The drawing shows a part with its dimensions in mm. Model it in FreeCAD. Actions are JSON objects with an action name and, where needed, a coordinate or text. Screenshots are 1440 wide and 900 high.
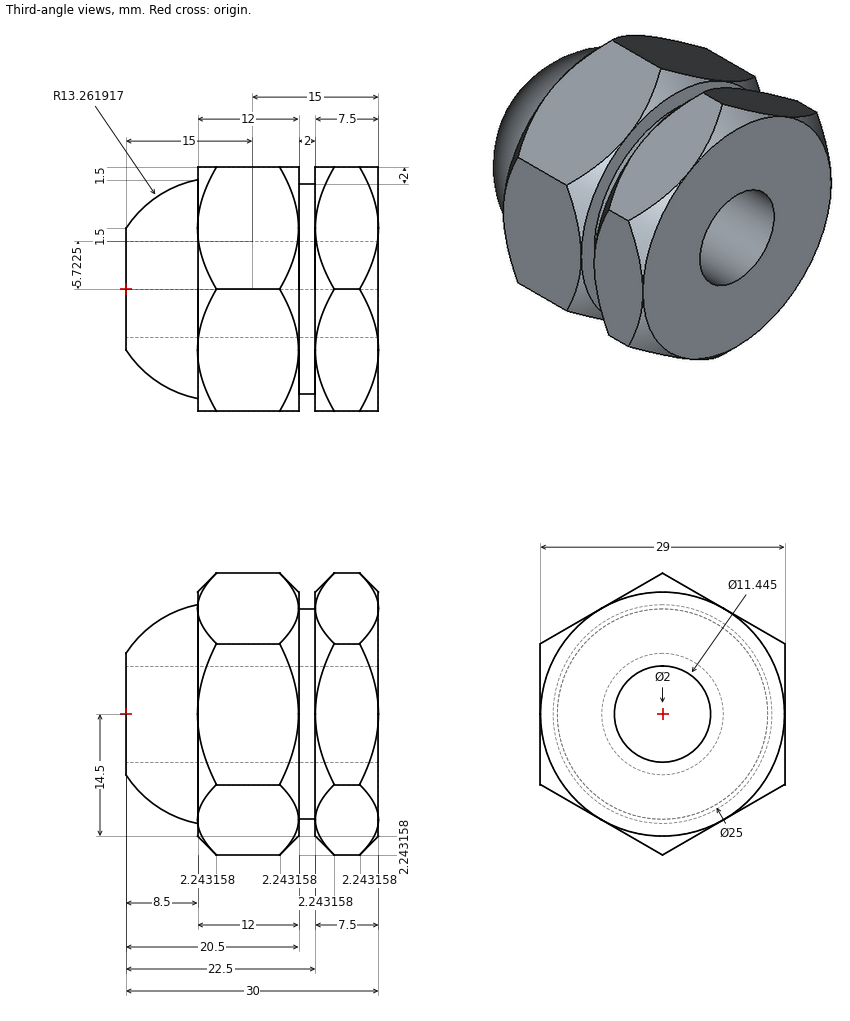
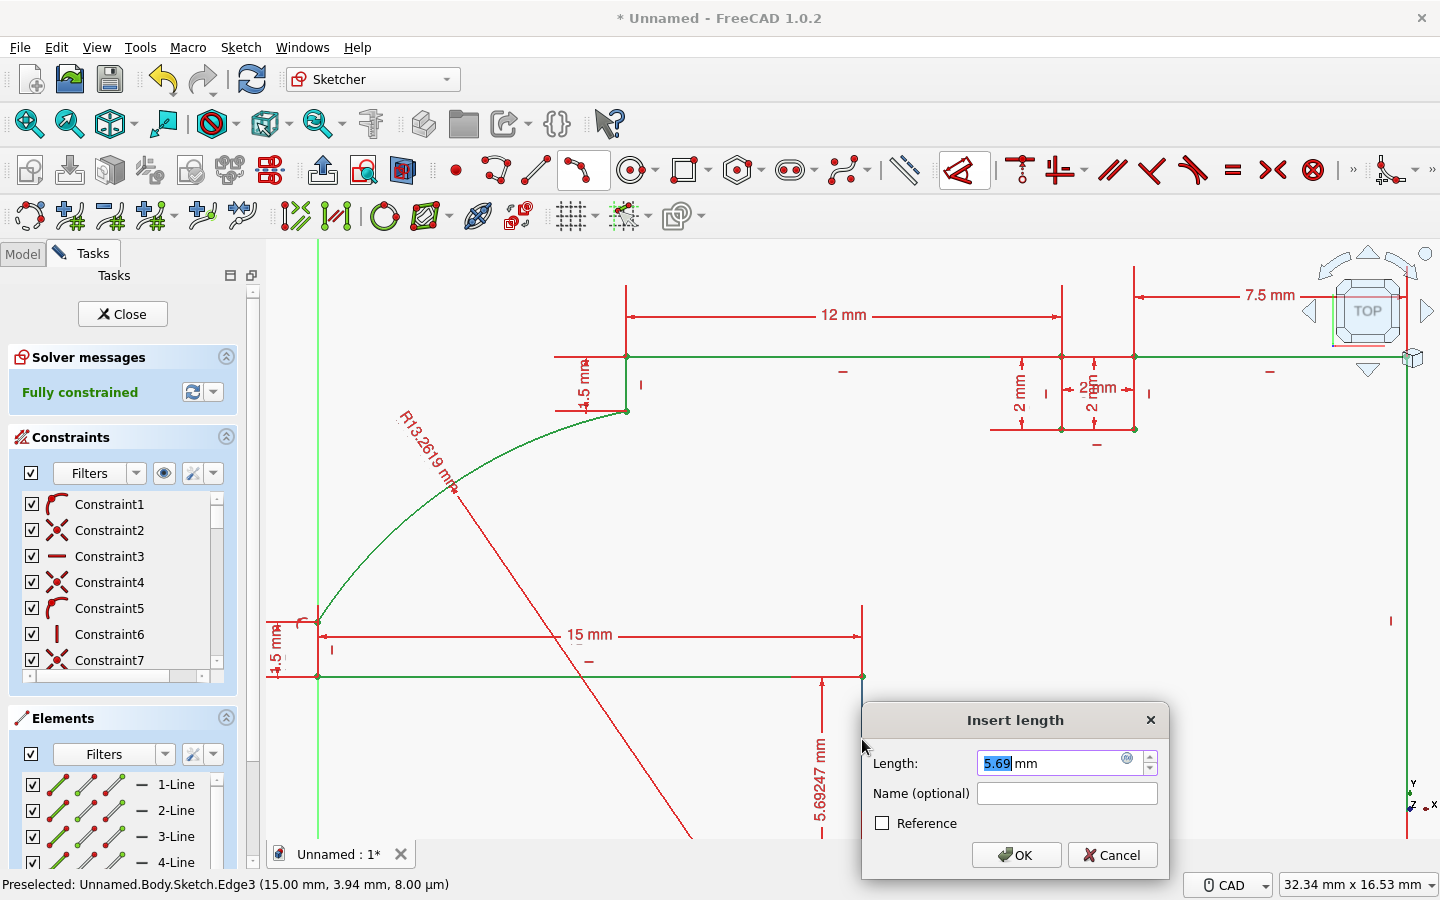
{"action": "type", "text": "5.7225"}
{"action": "key", "text": "Return"}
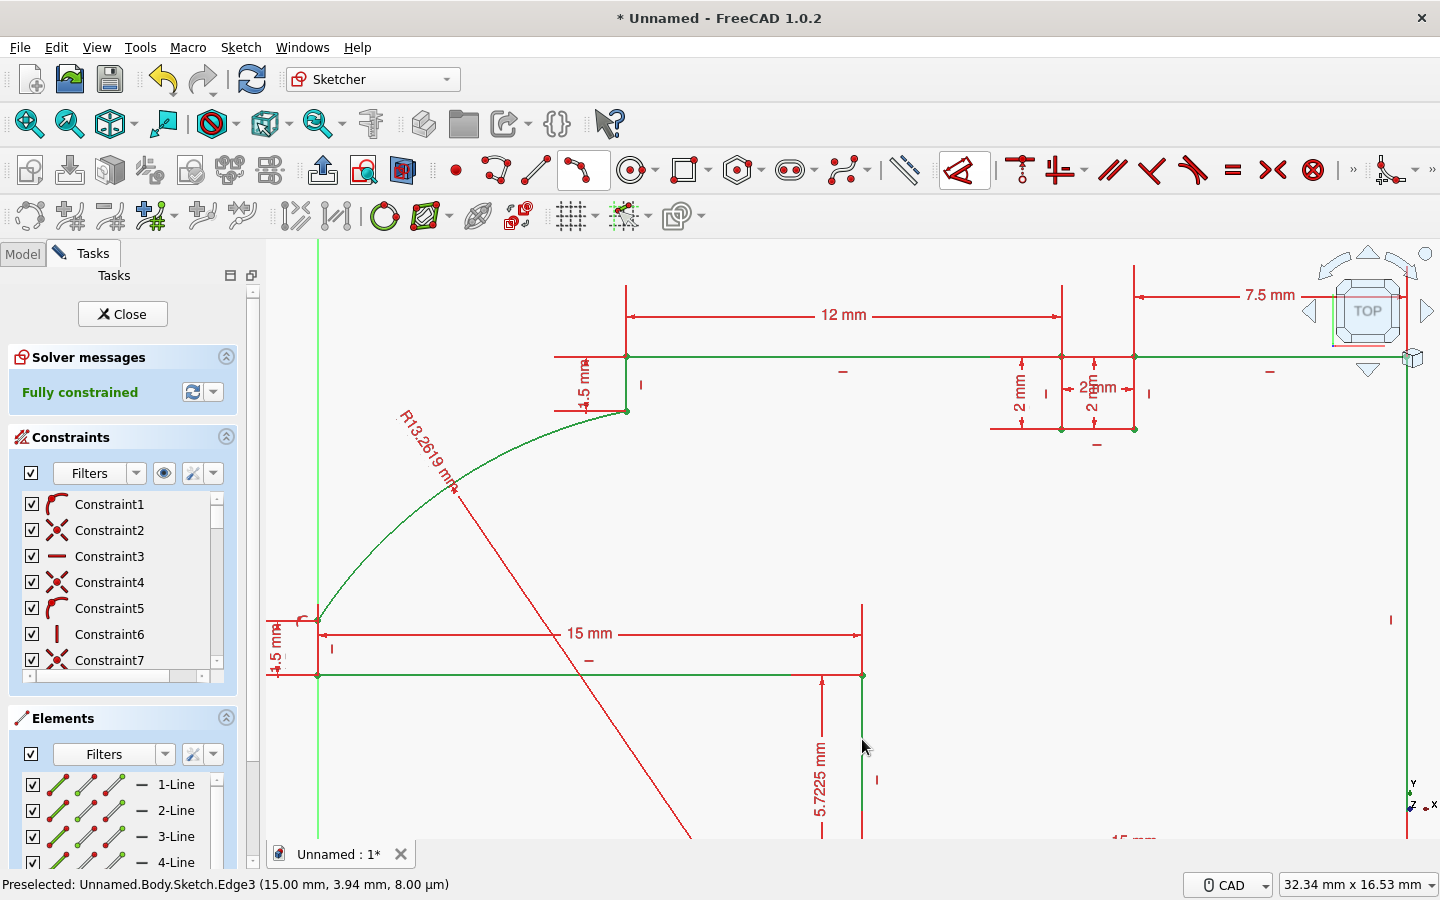
{"action": "left_click", "coordinate": [123, 314]}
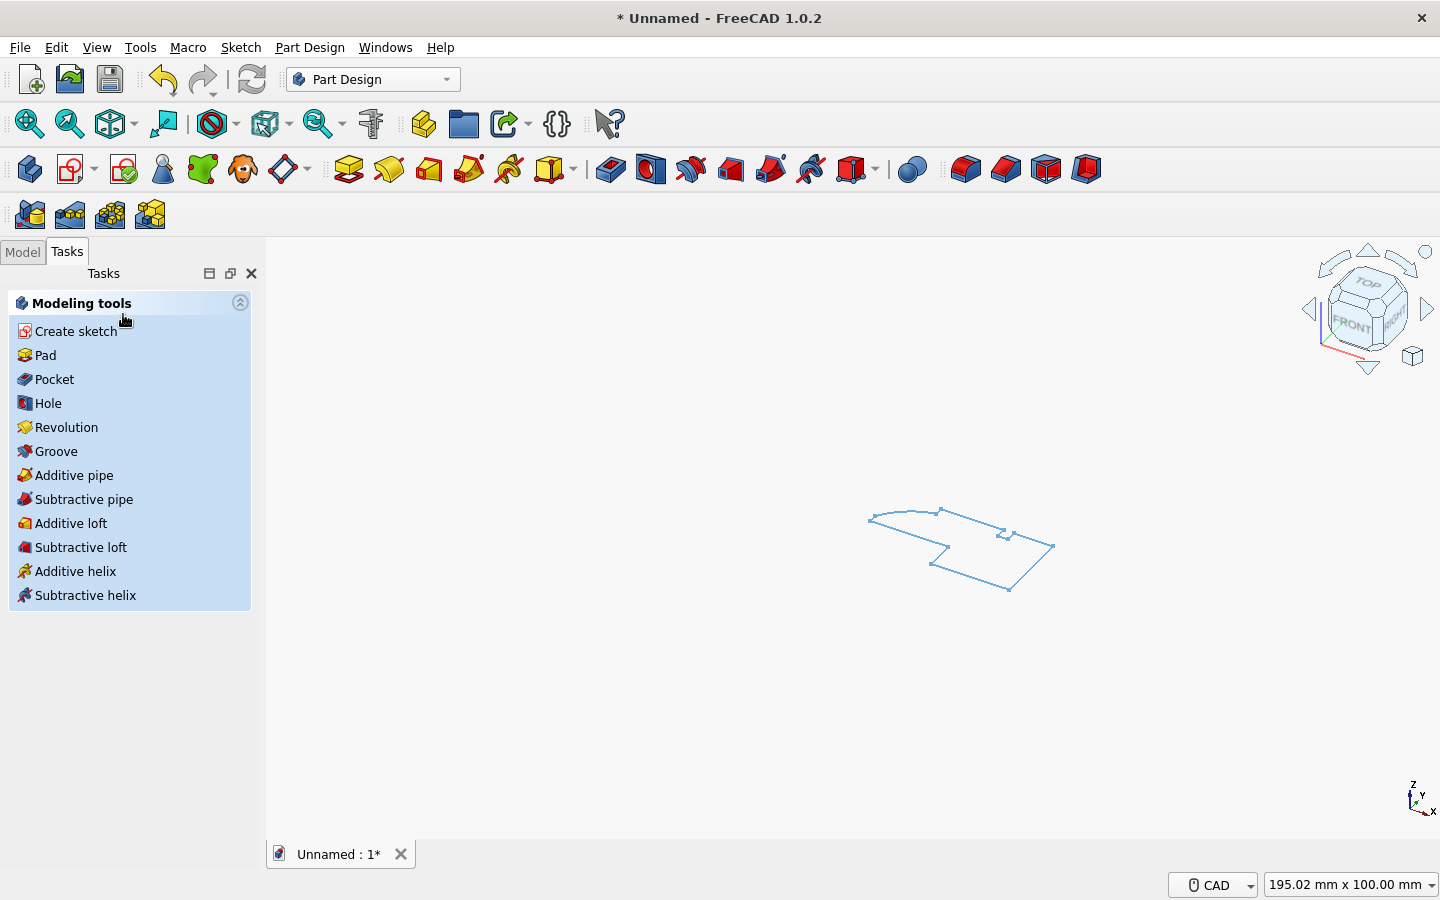
{"action": "left_click", "coordinate": [390, 170]}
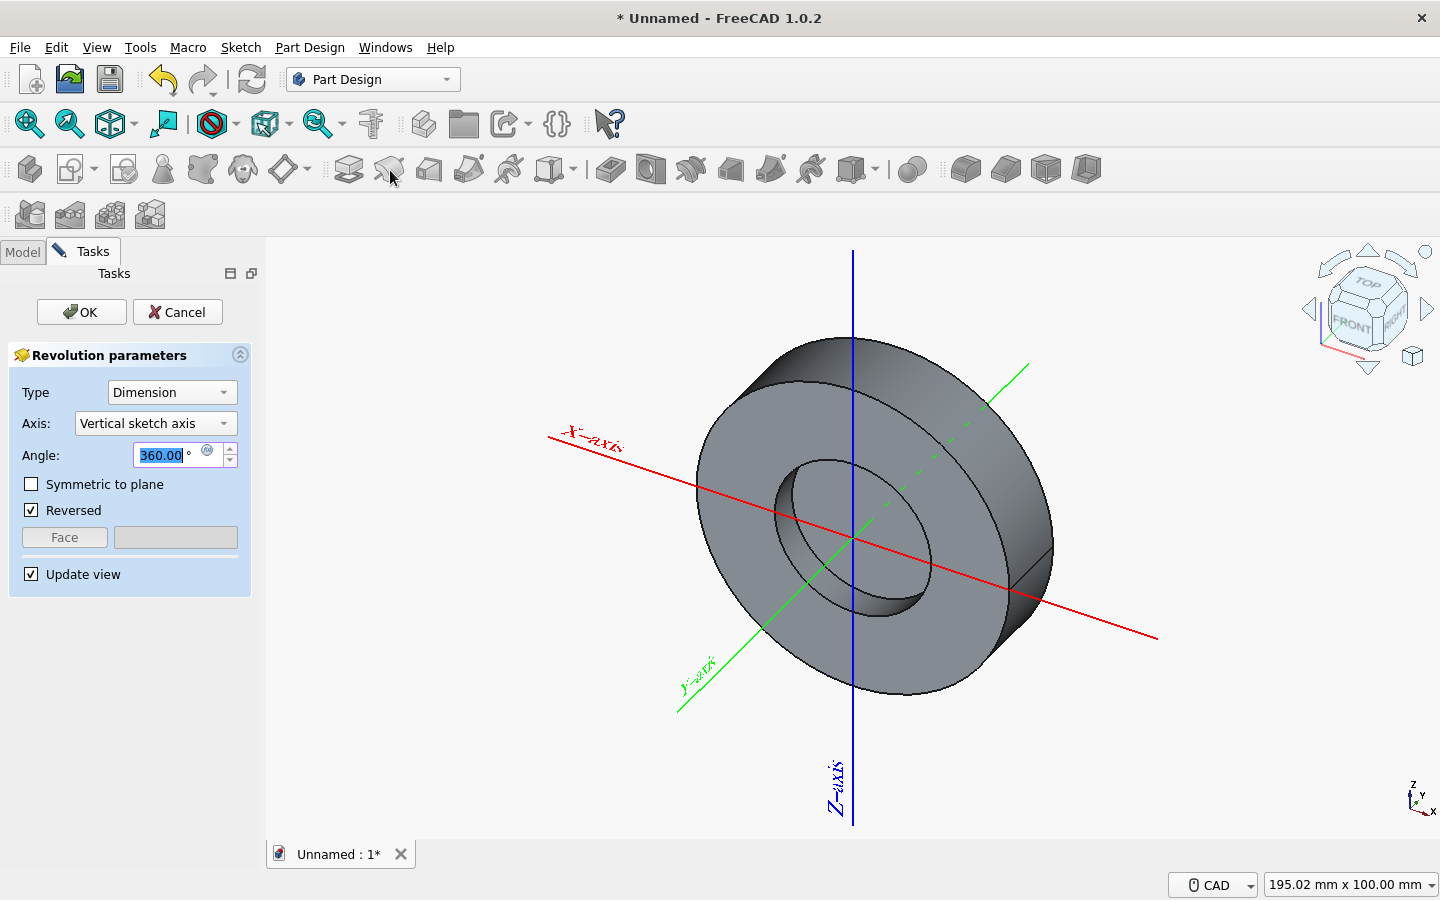
{"action": "left_click", "coordinate": [156, 424]}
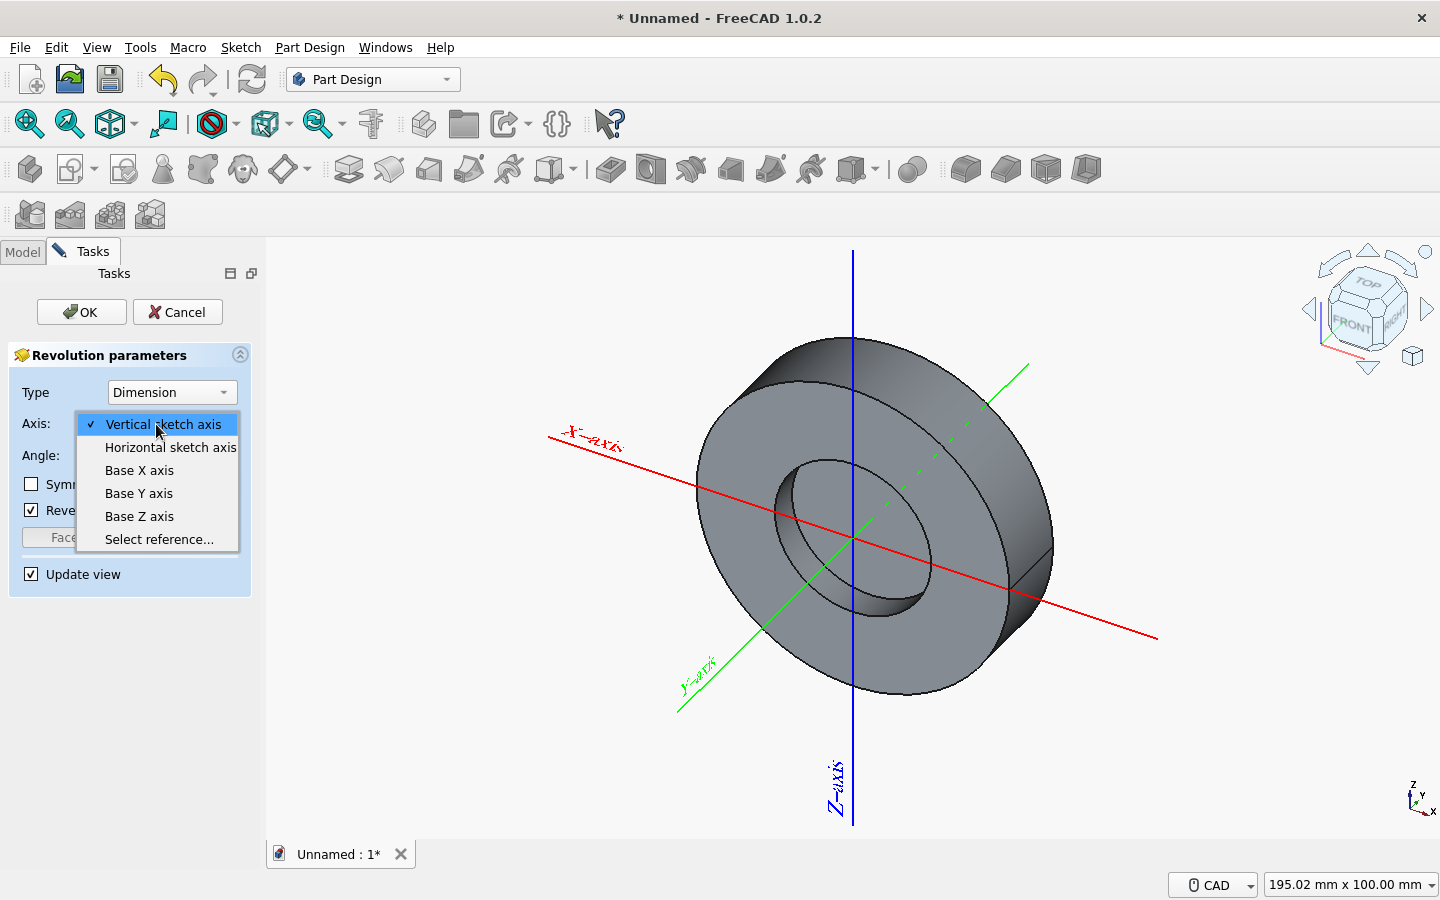
{"action": "left_click", "coordinate": [156, 448]}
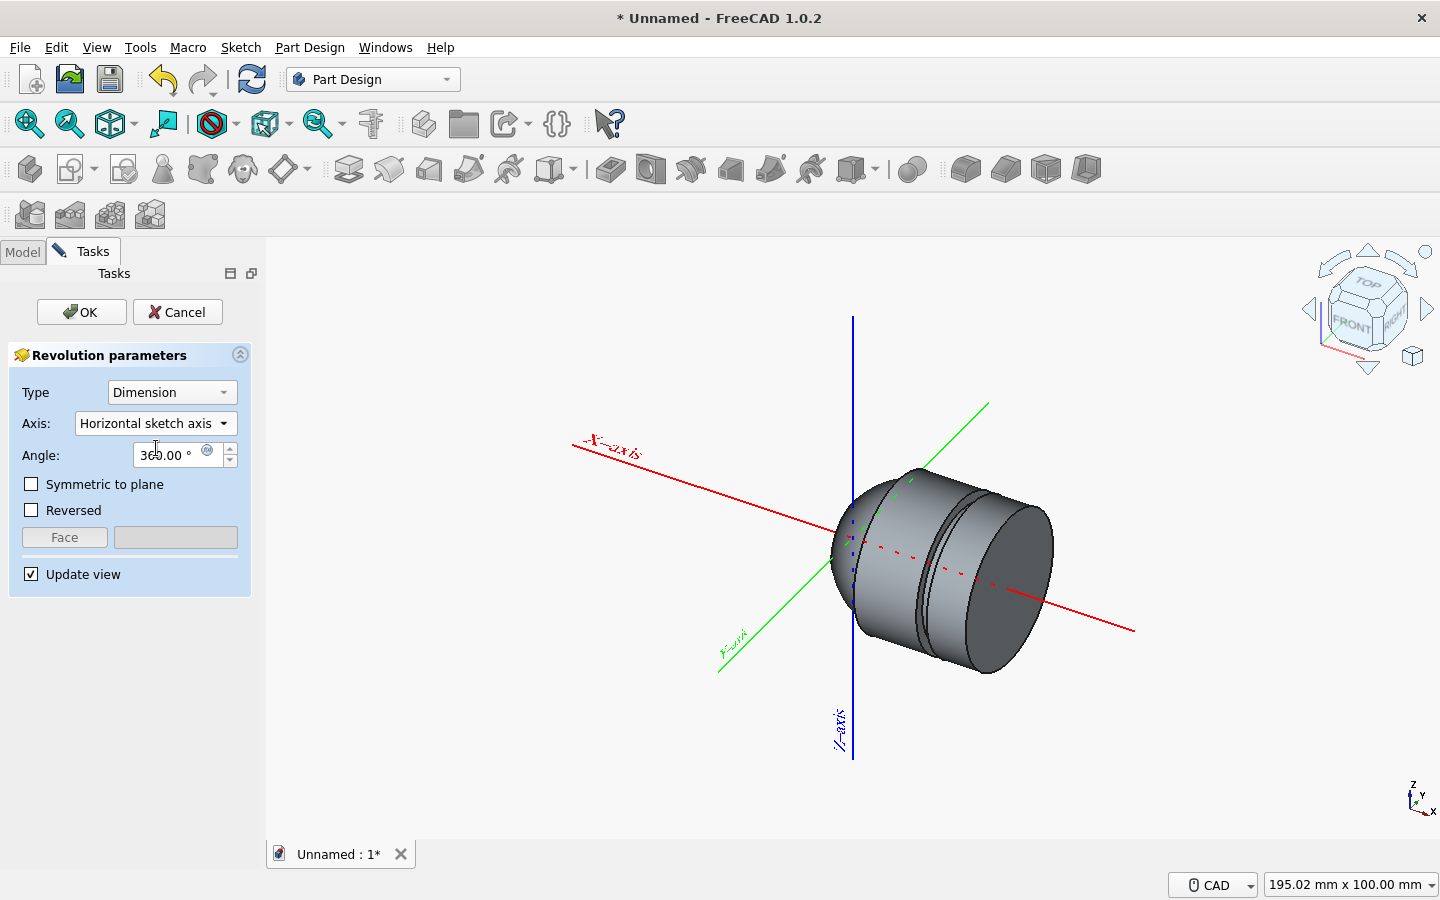
{"action": "left_click", "coordinate": [82, 312]}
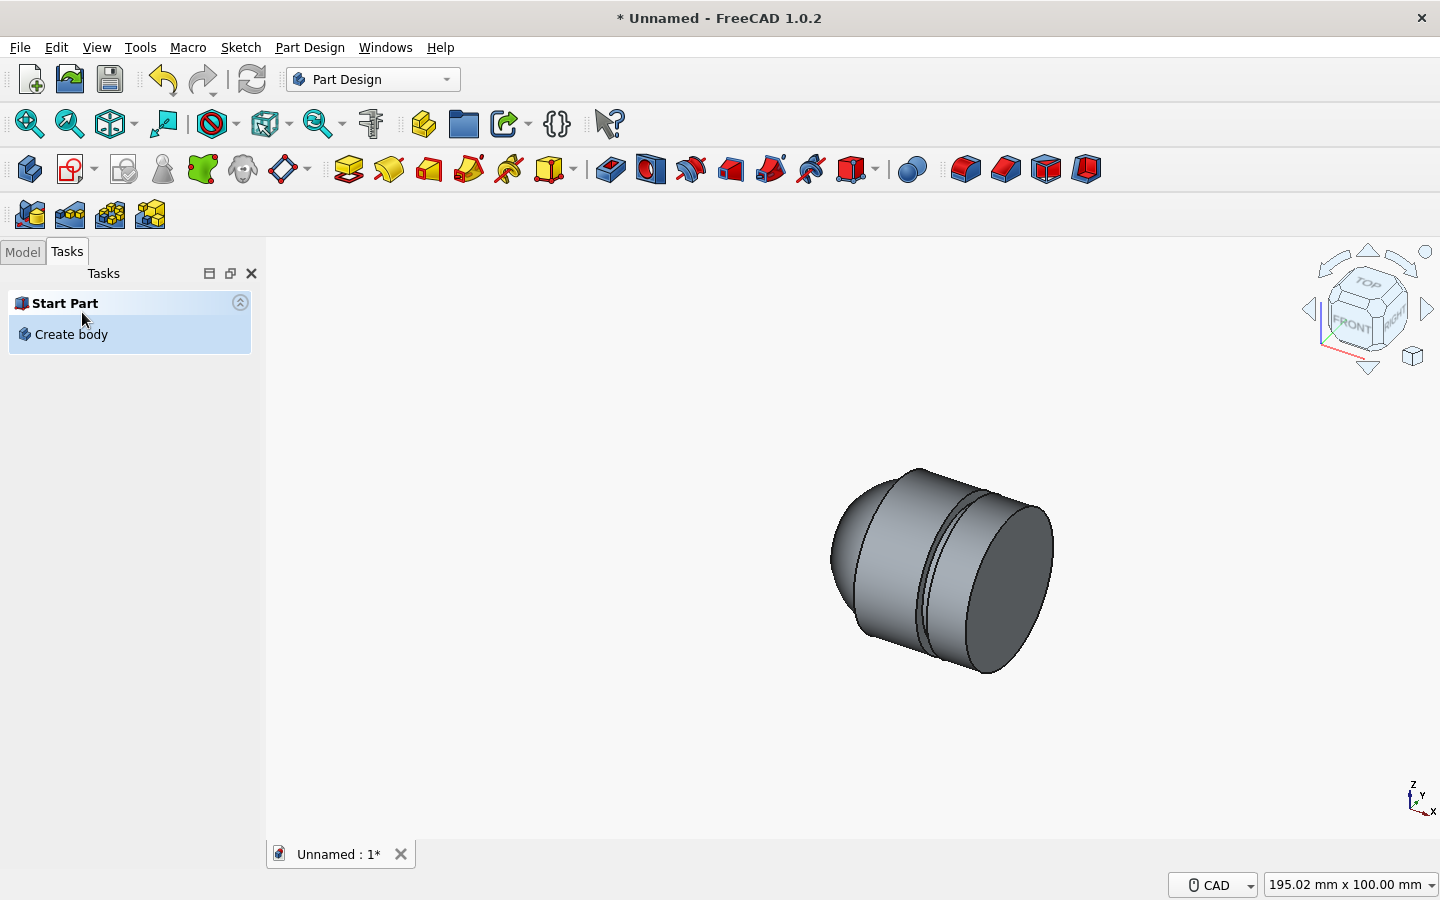
{"action": "left_click", "coordinate": [23, 251]}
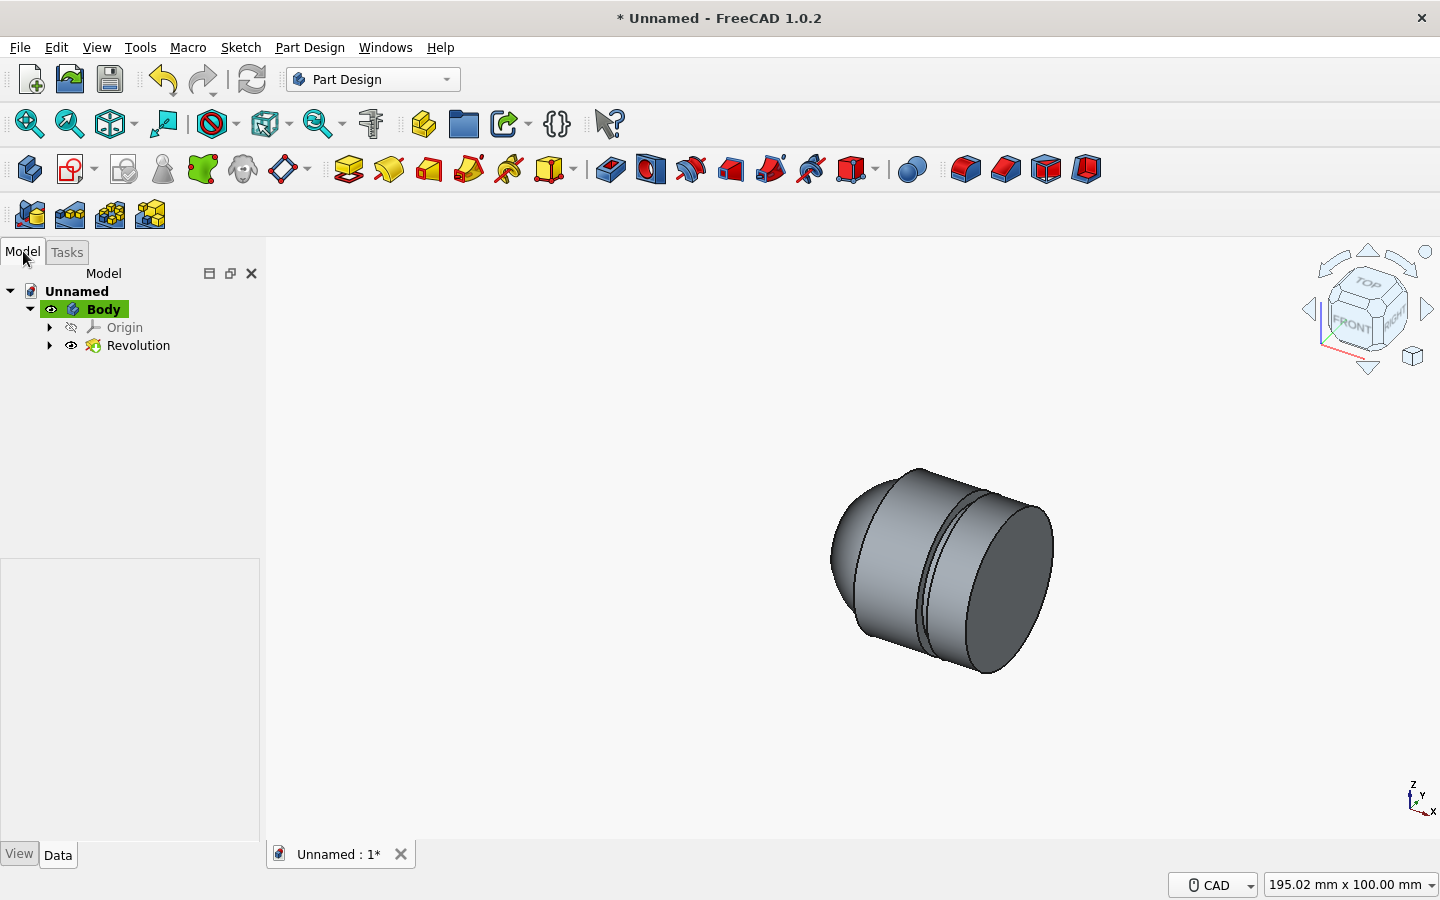
{"action": "left_click", "coordinate": [50, 327]}